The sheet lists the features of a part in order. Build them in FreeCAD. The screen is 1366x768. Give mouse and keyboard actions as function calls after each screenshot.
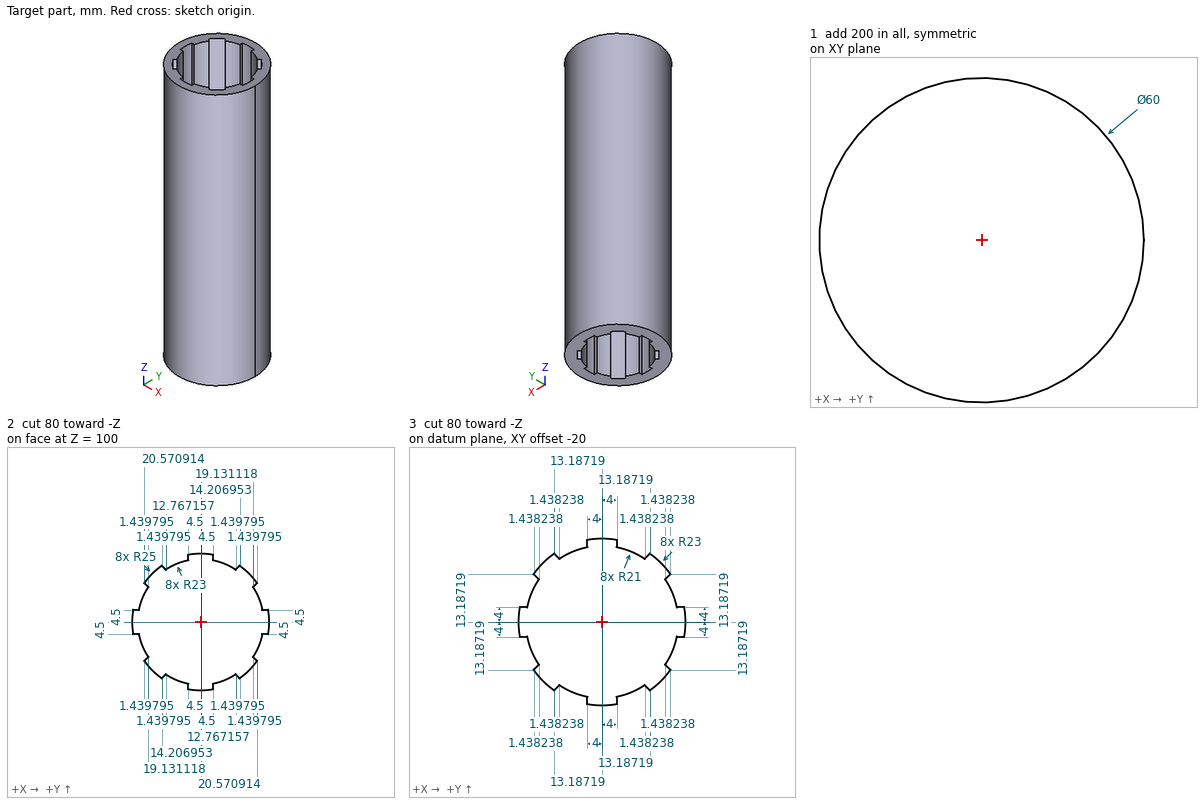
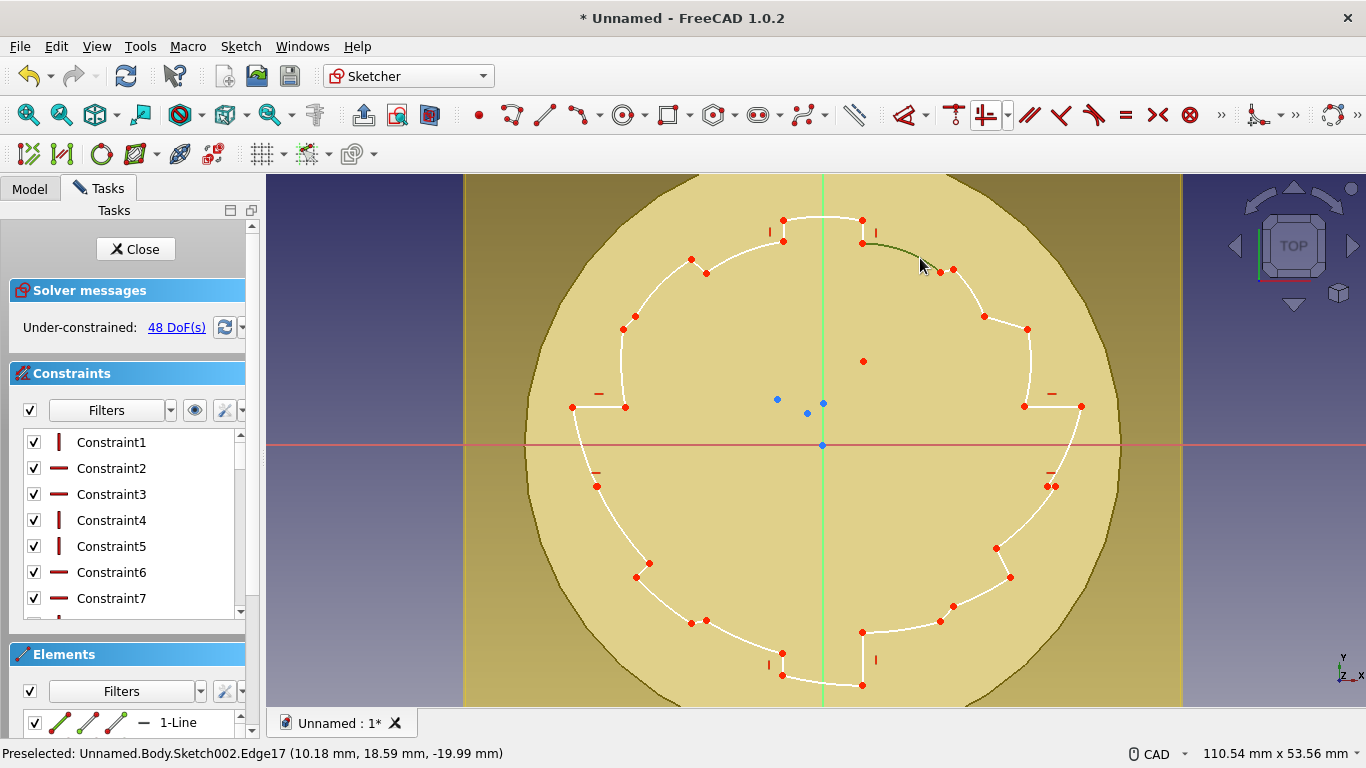
click(672, 274)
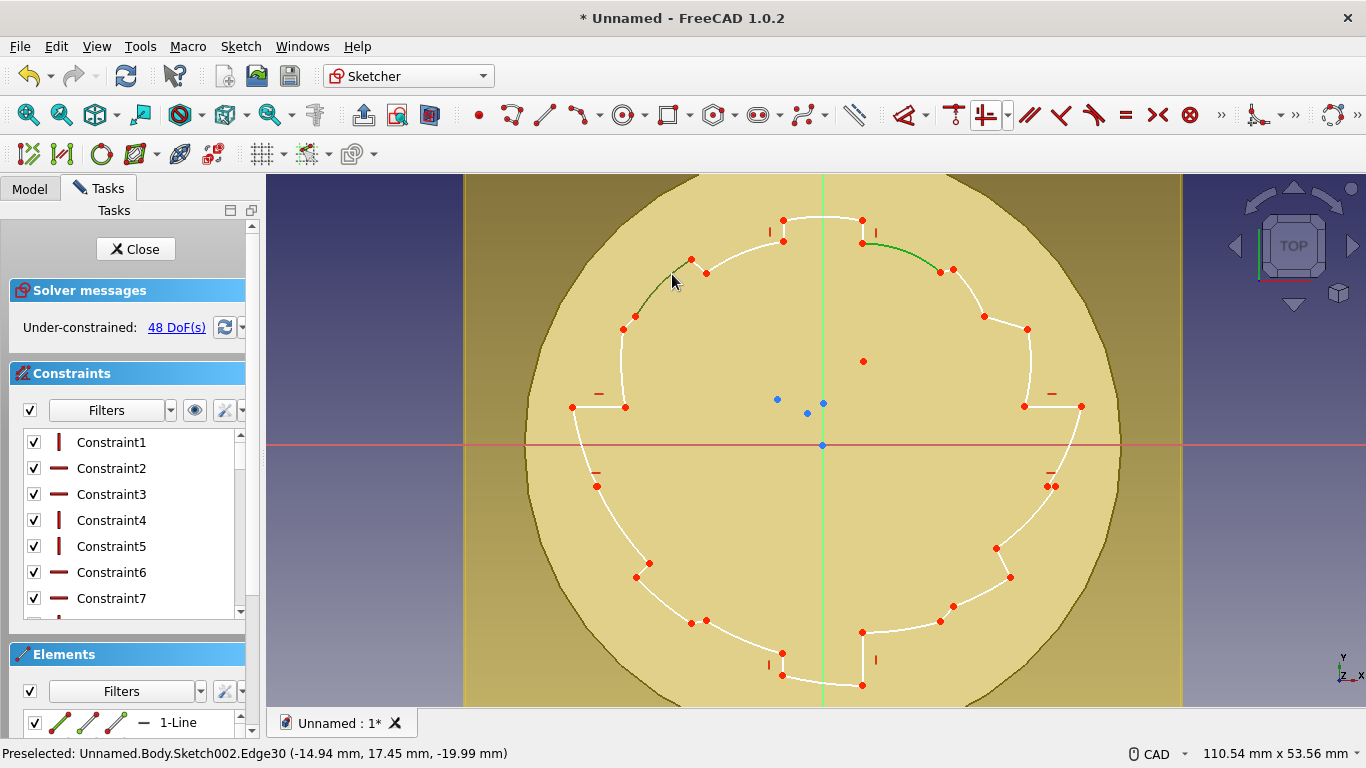
click(954, 116)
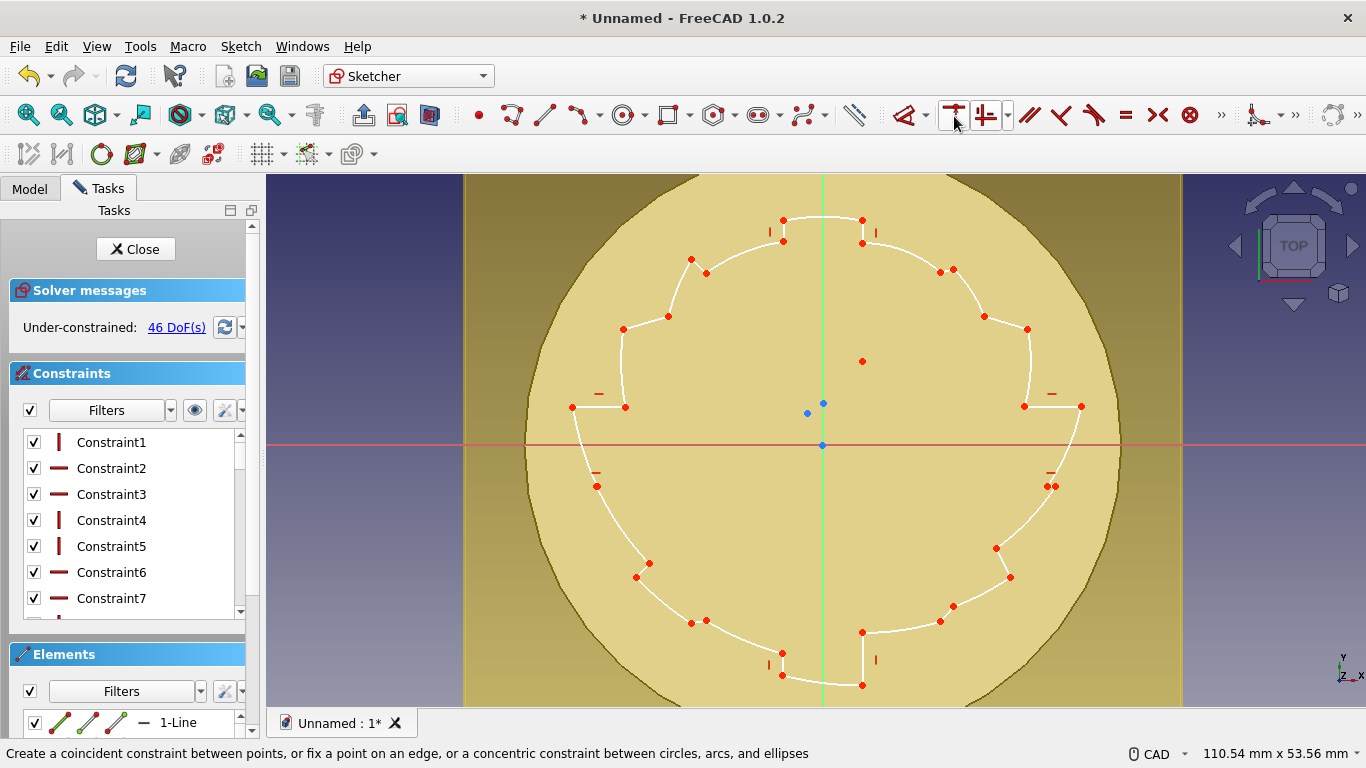
click(920, 258)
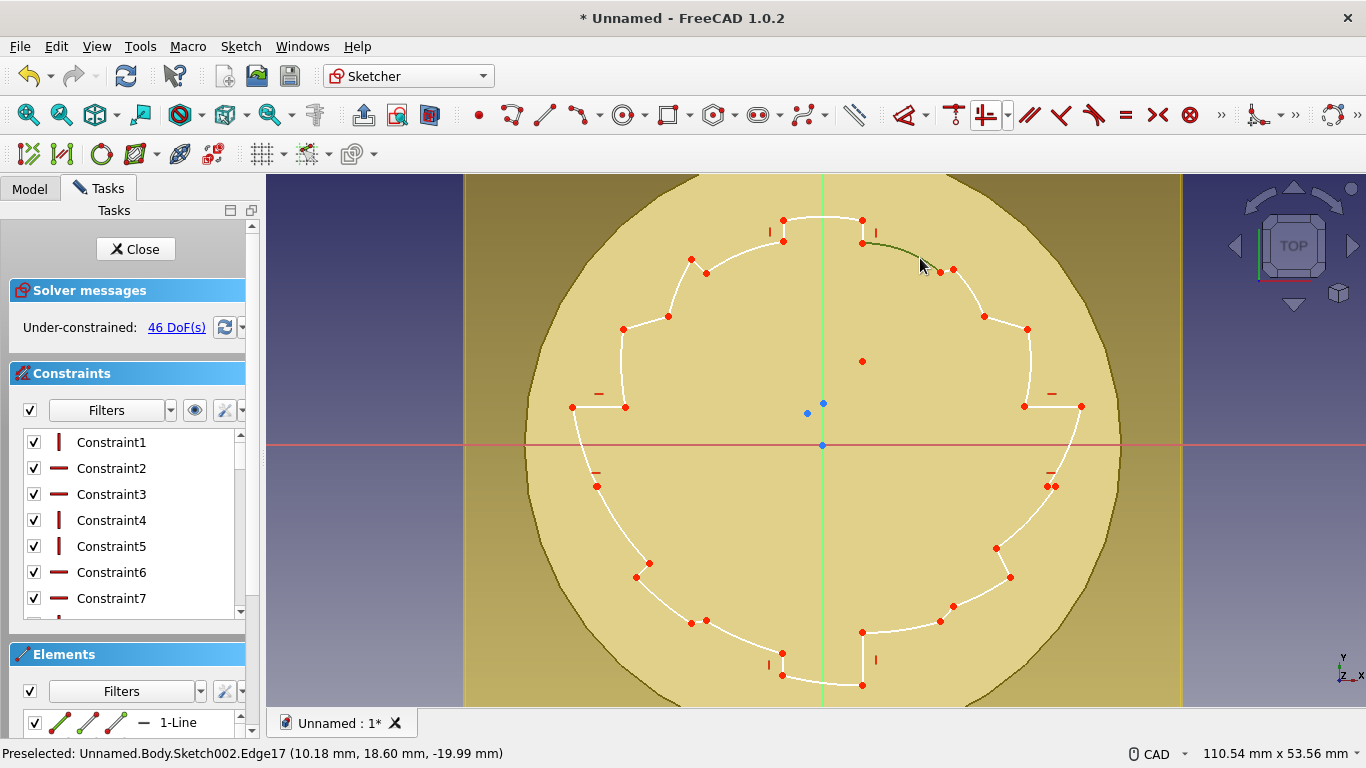
click(759, 247)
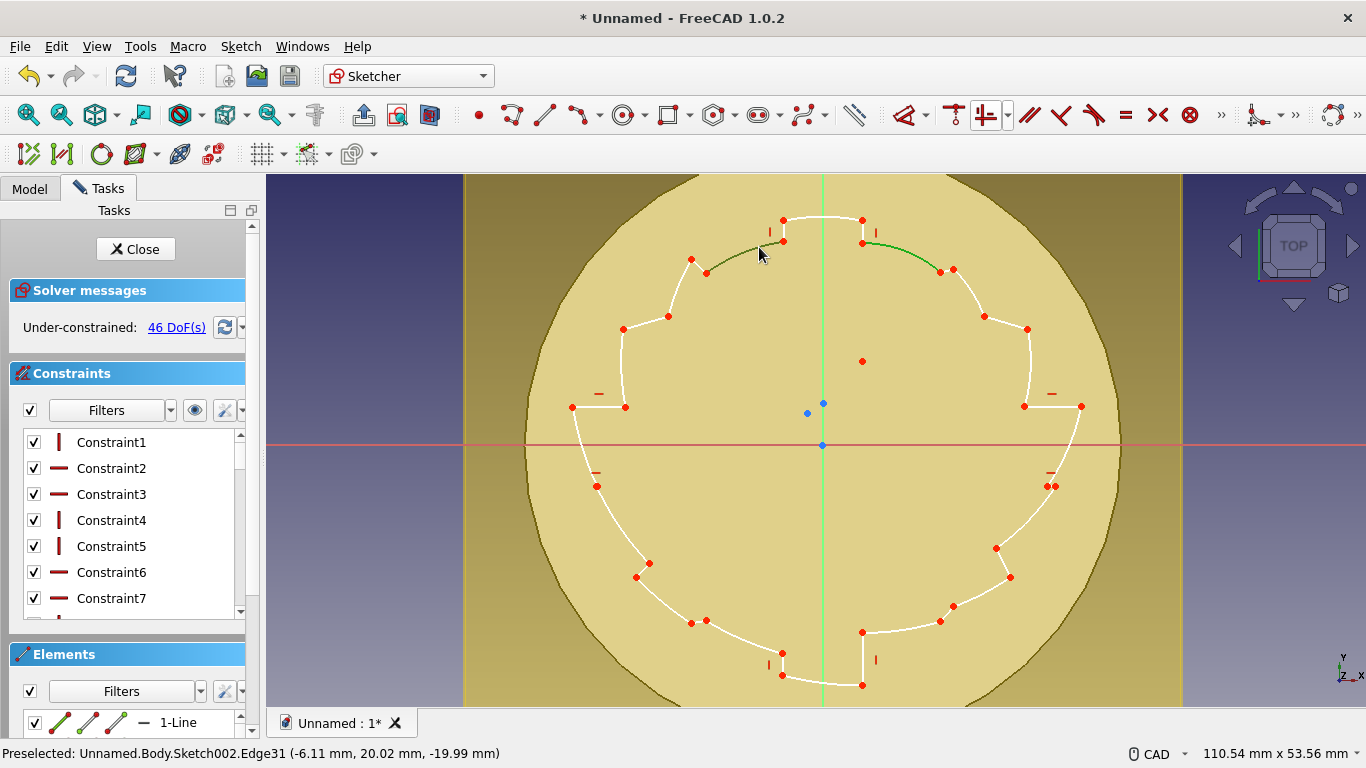
click(954, 116)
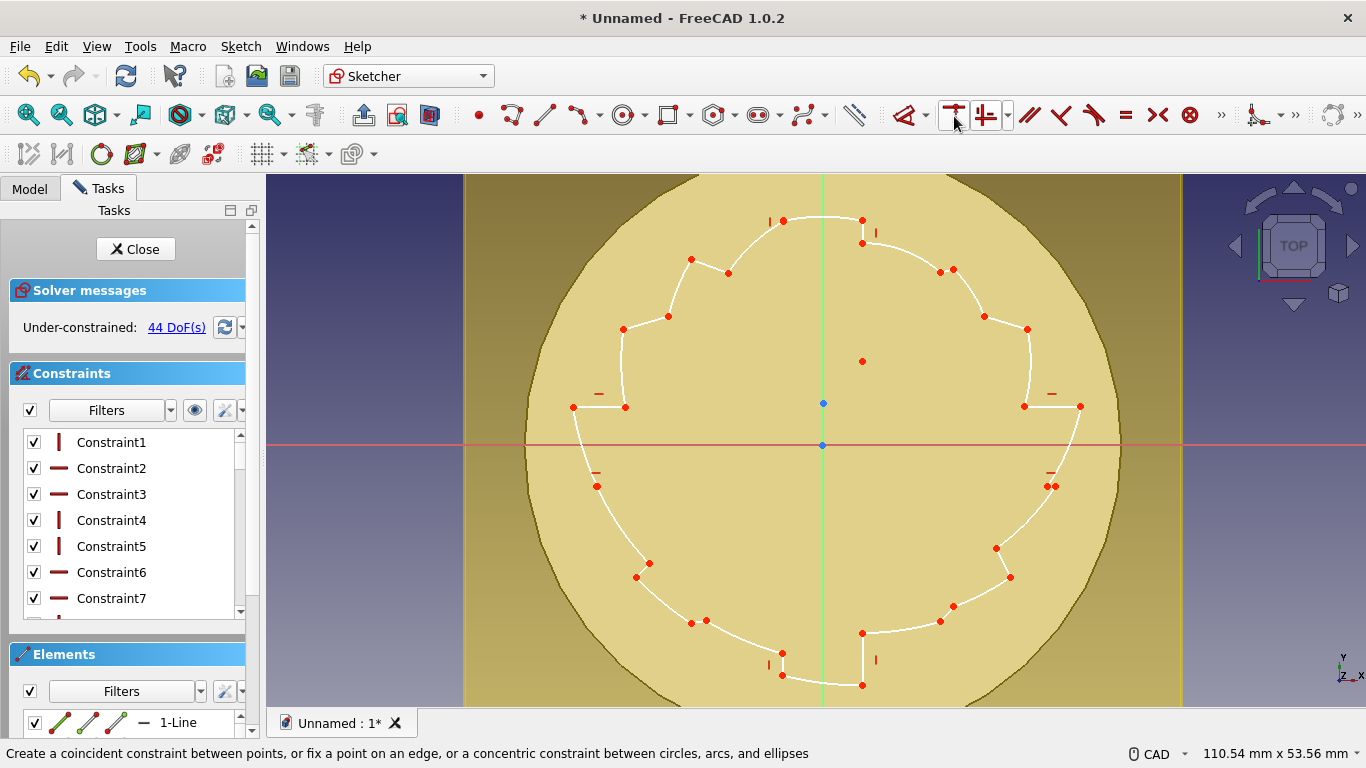
click(920, 258)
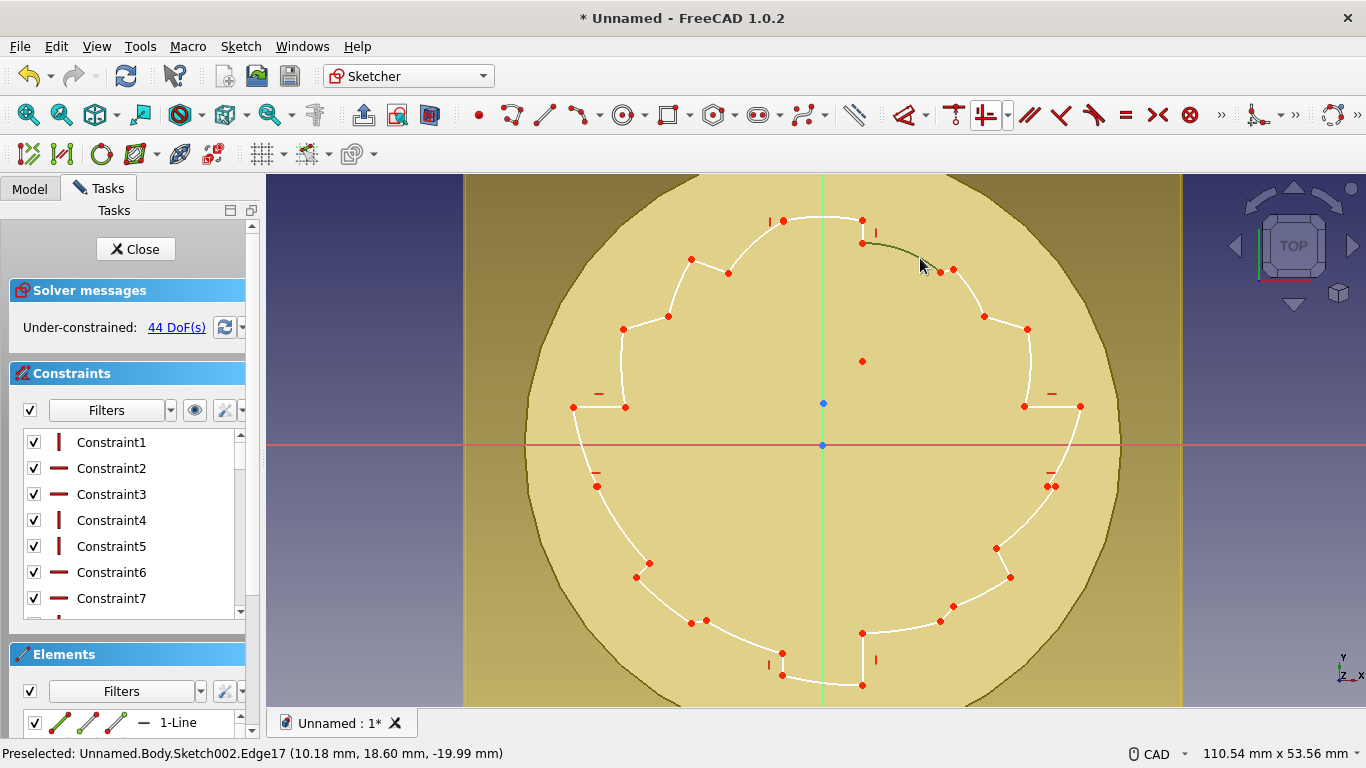
click(839, 217)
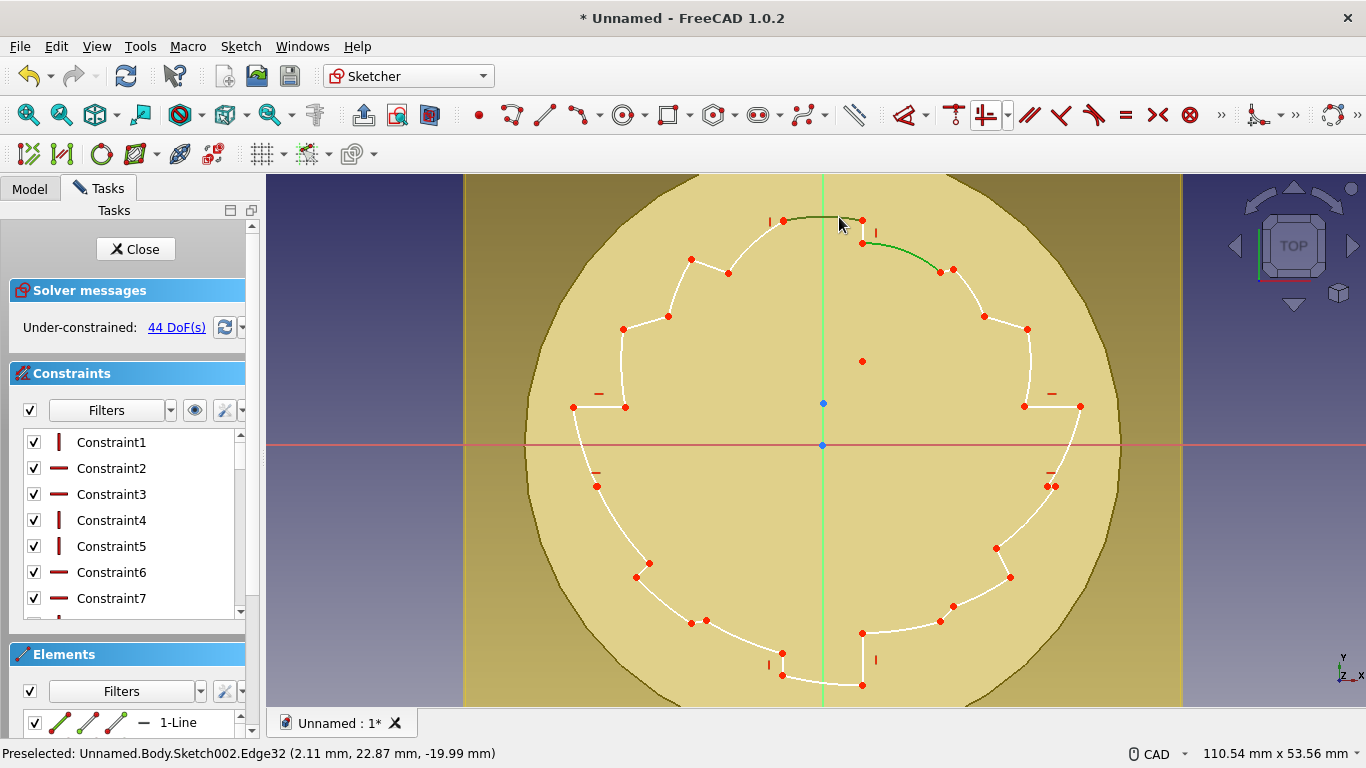
click(954, 116)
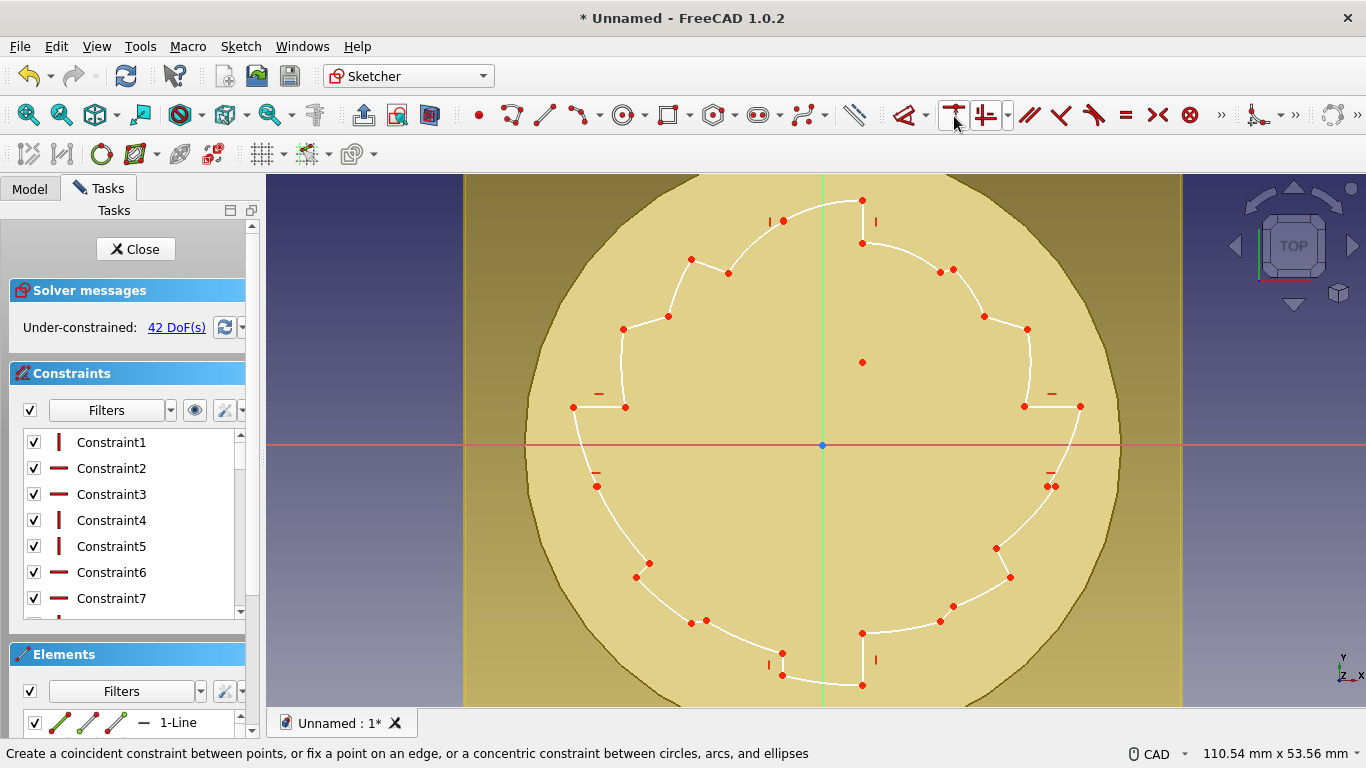
drag(813, 352, 872, 455)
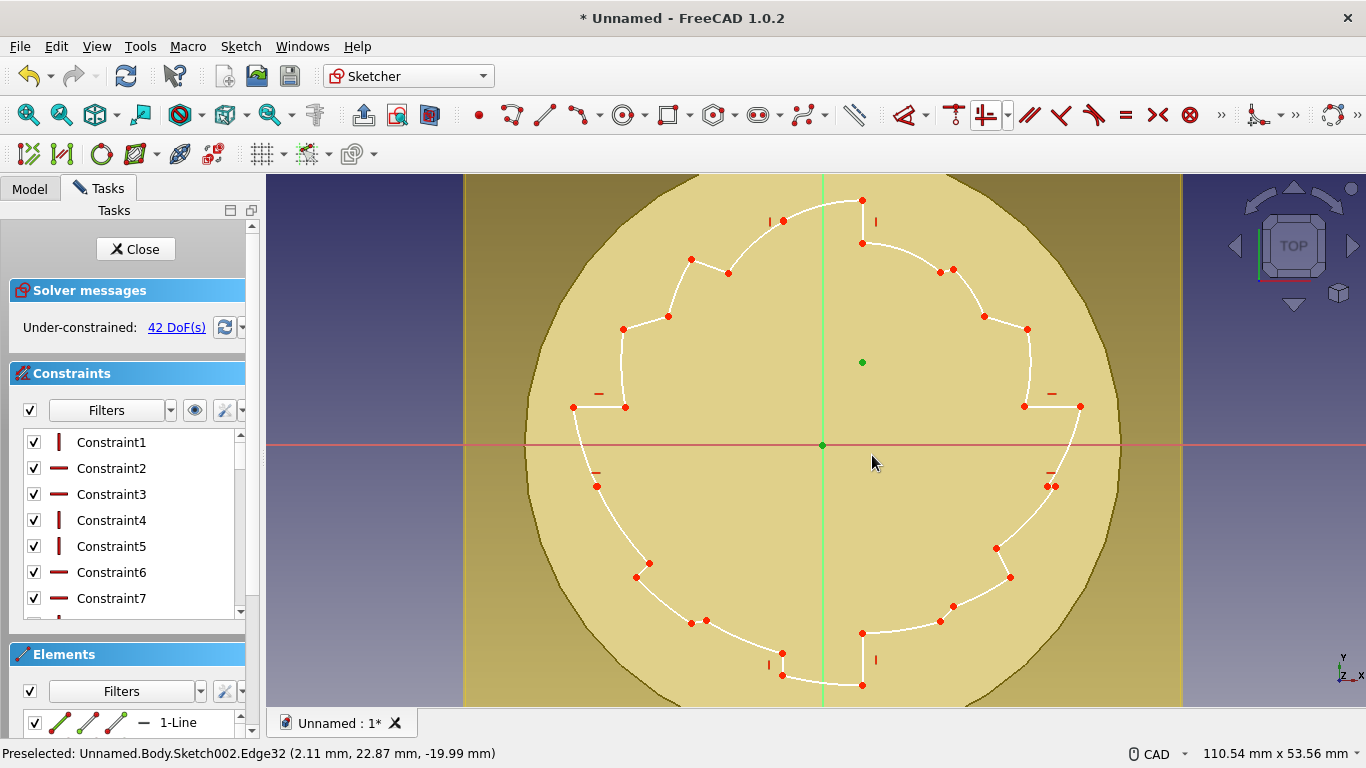
click(954, 116)